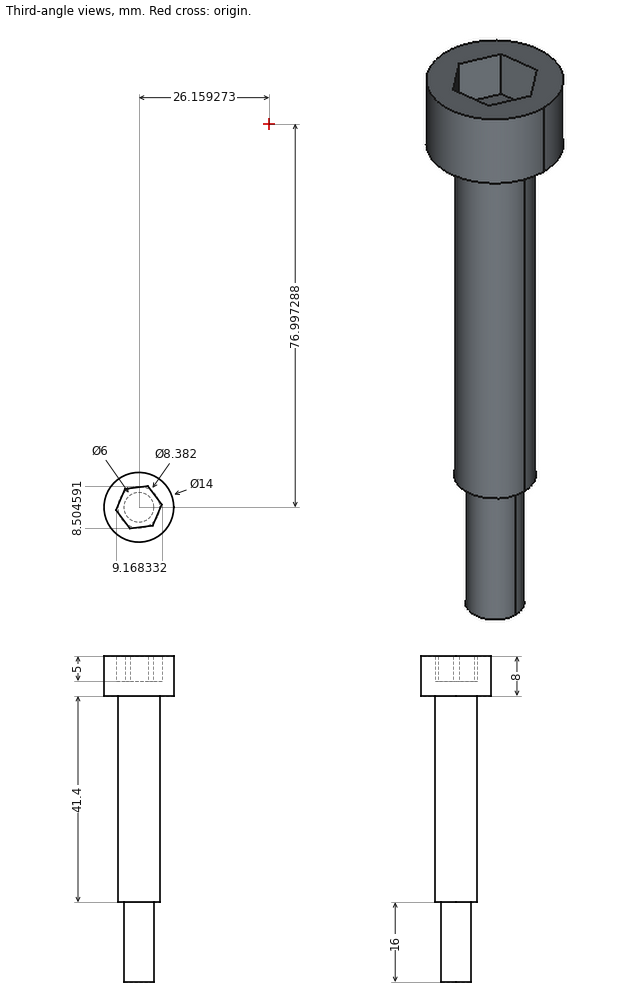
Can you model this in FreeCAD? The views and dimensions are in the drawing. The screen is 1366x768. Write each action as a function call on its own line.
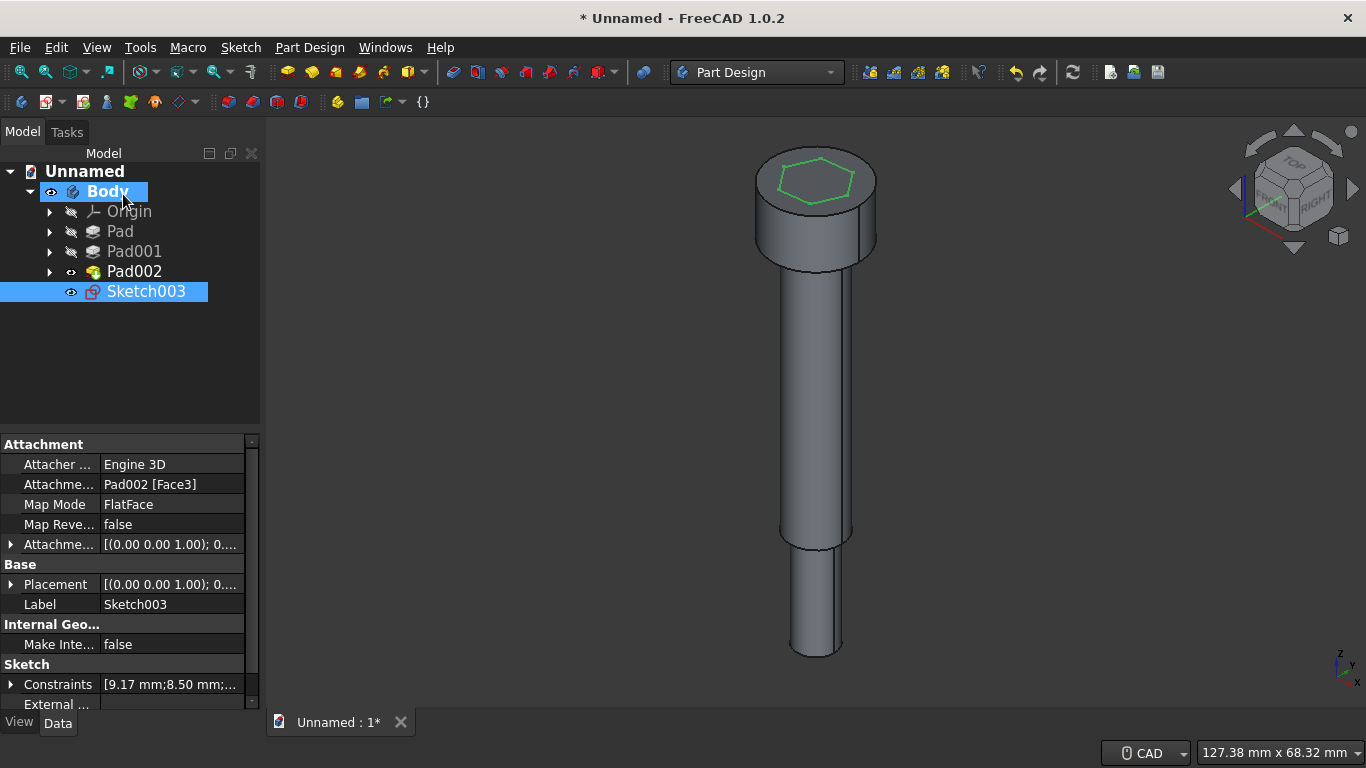
click(454, 72)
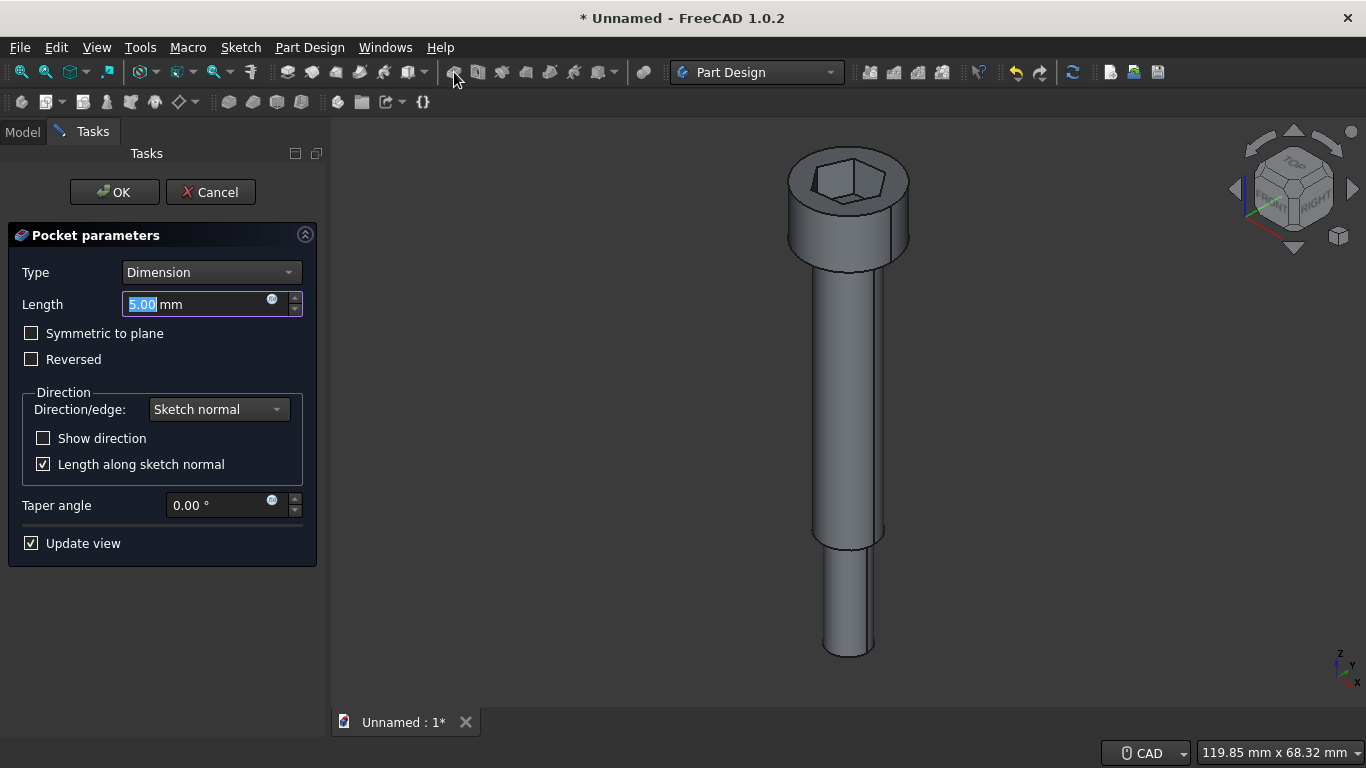
text(5)
key(Tab)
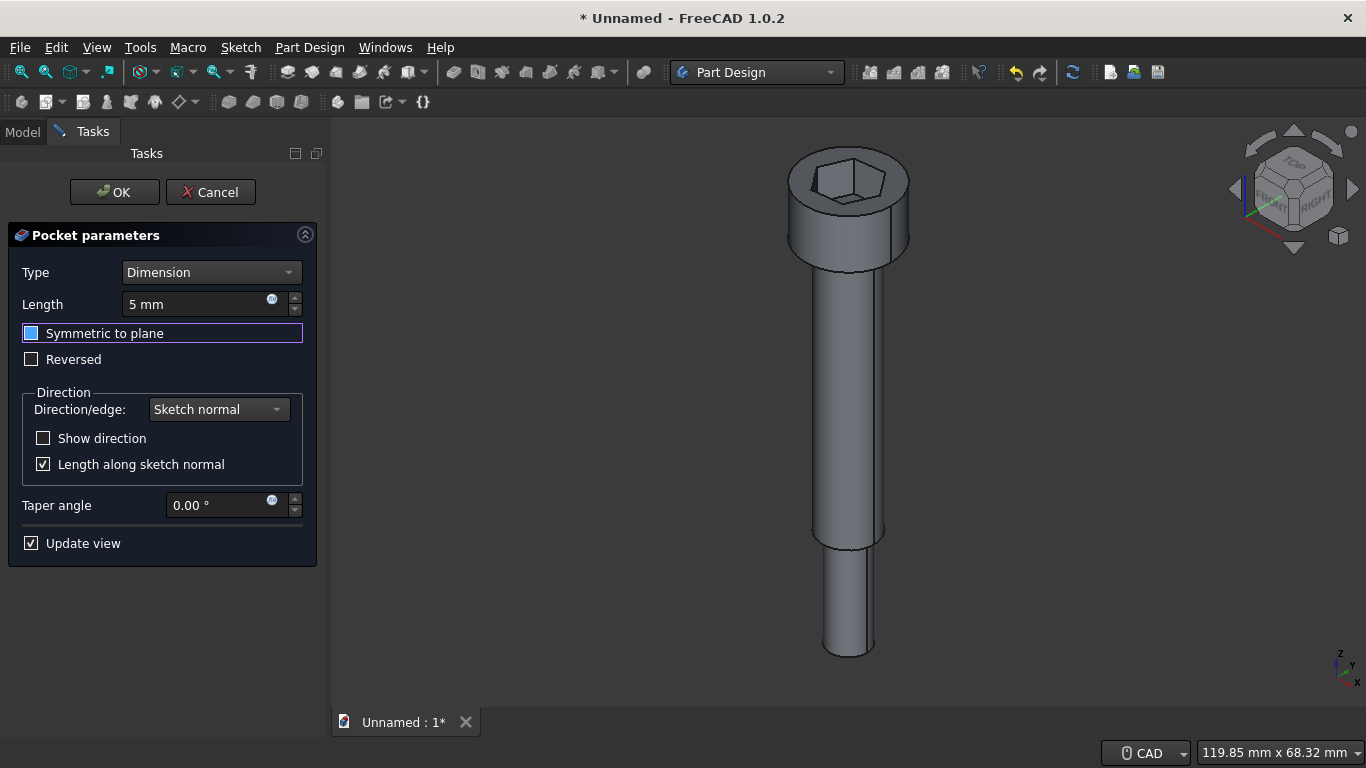
click(115, 192)